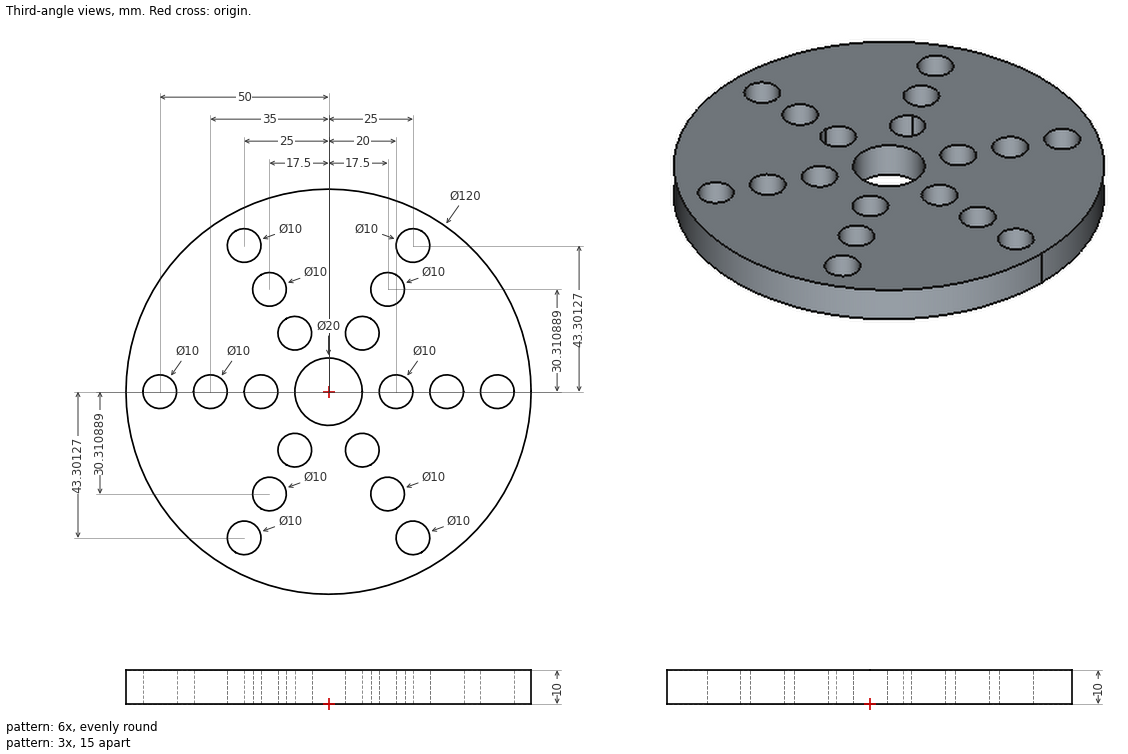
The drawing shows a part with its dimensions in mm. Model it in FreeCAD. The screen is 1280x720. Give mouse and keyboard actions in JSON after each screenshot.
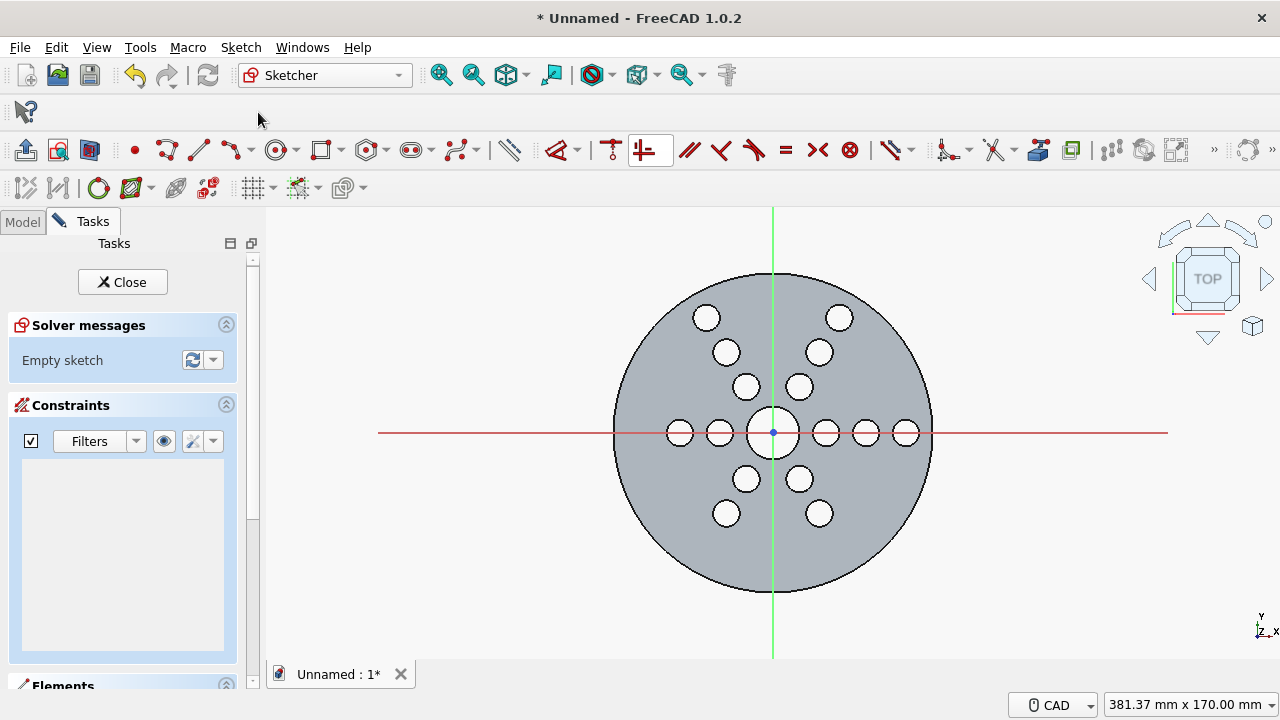
{"action": "scroll", "coordinate": [634, 433], "scroll_direction": "up", "scroll_amount": 12}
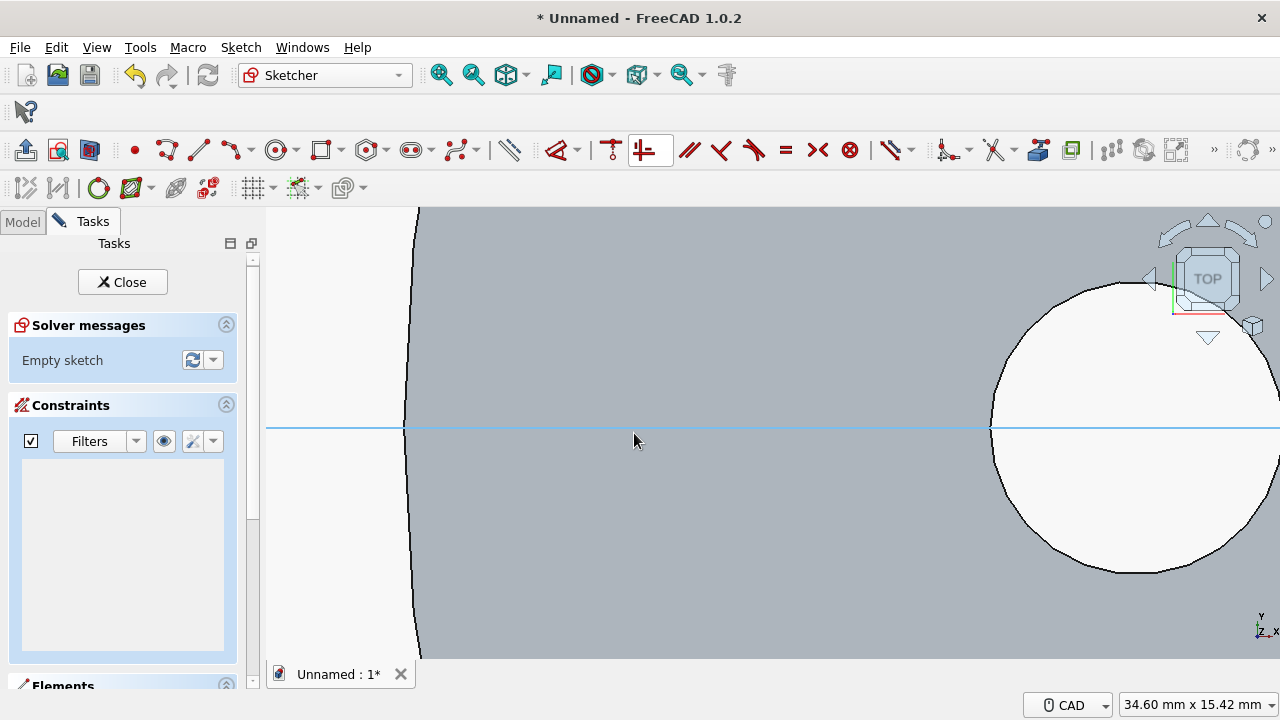
{"action": "key", "text": "g c"}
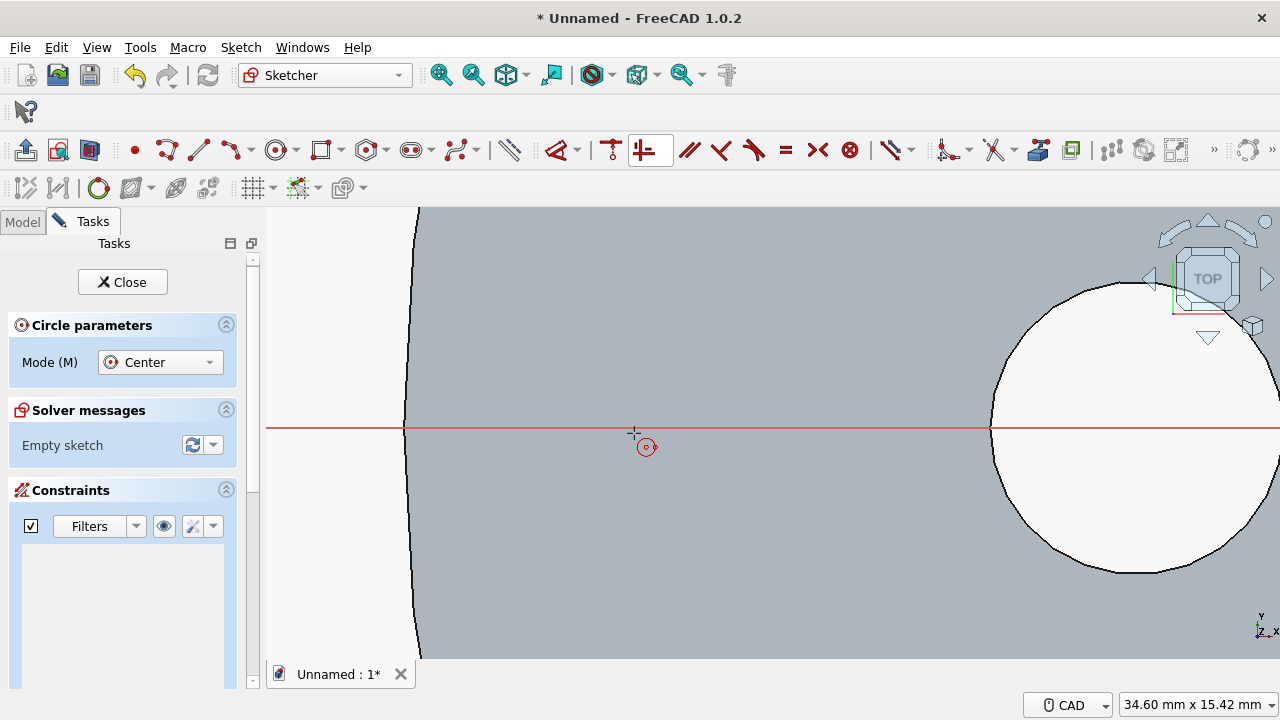
{"action": "left_click", "coordinate": [697, 428]}
{"action": "left_click", "coordinate": [801, 324]}
{"action": "key", "text": "Escape"}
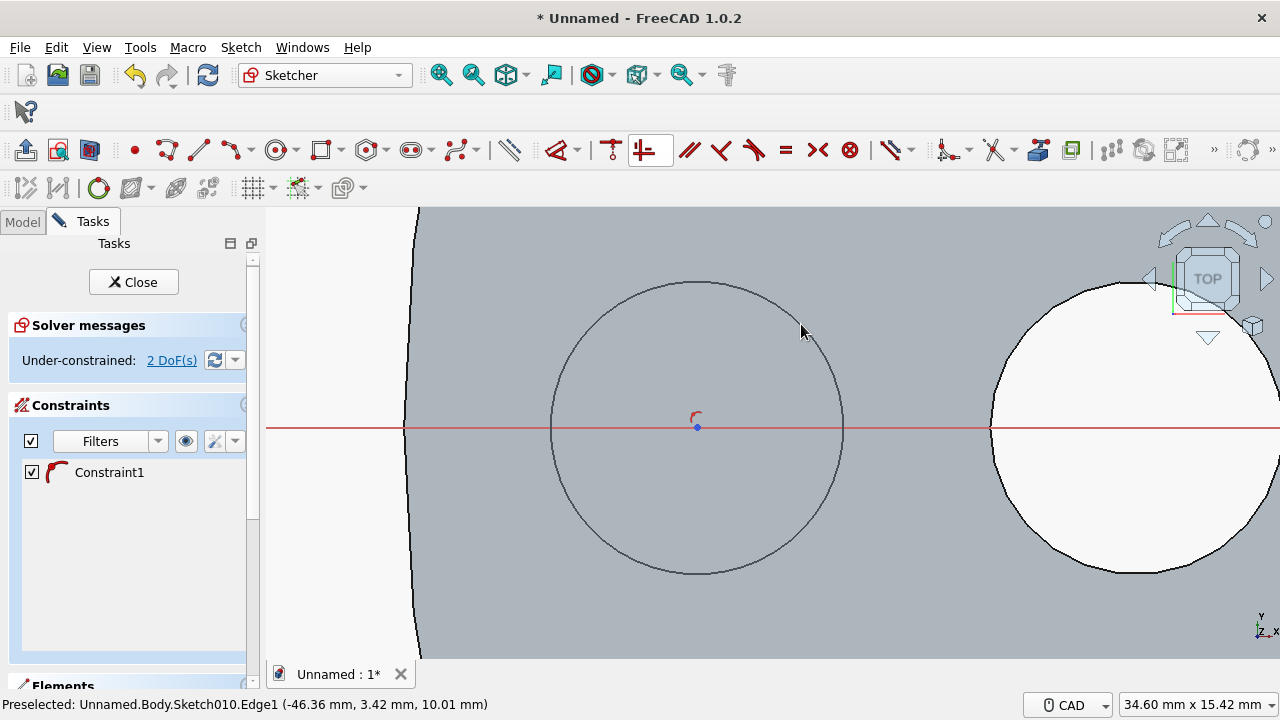
{"action": "left_click", "coordinate": [556, 150]}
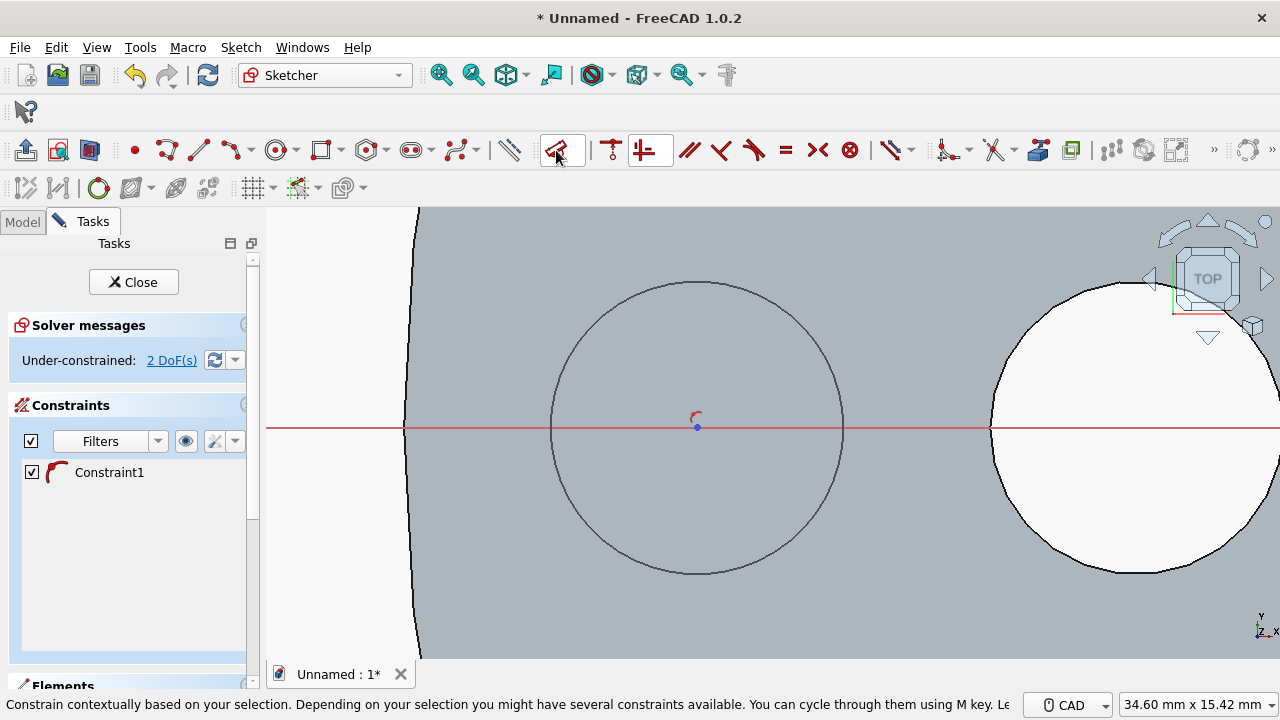
{"action": "left_click", "coordinate": [800, 324]}
{"action": "left_click", "coordinate": [823, 301]}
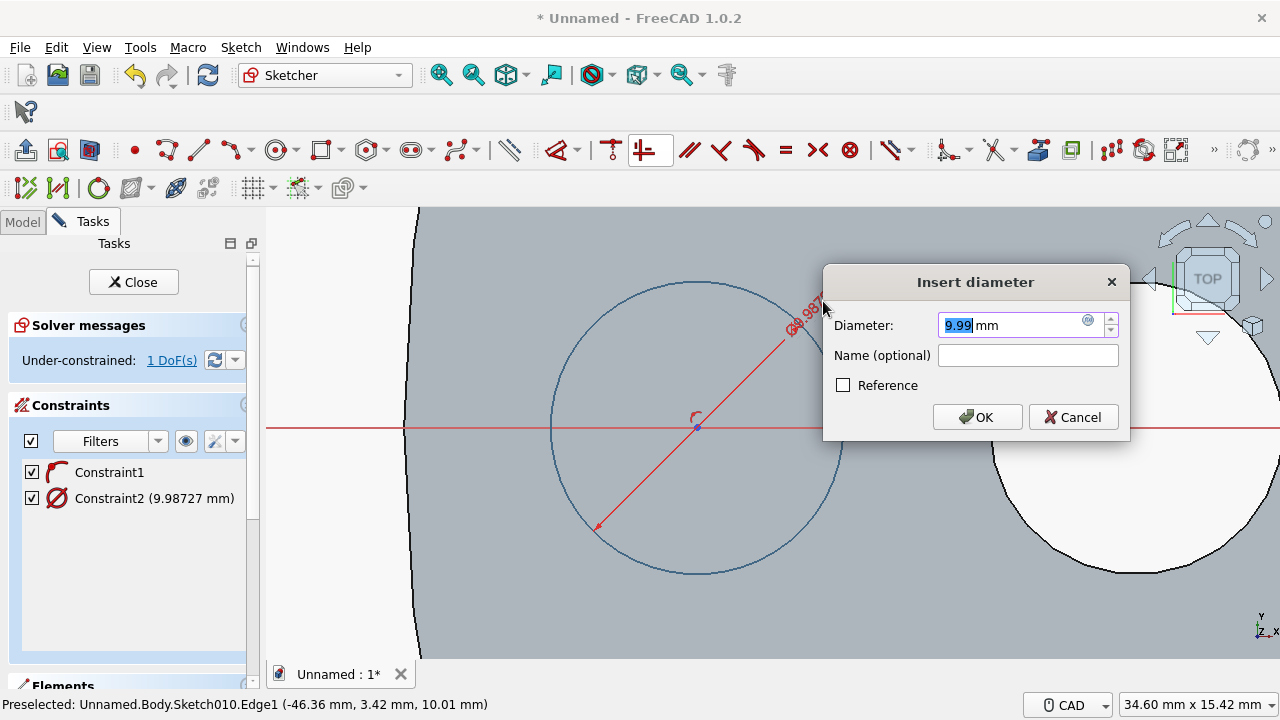
{"action": "type", "text": "10"}
{"action": "key", "text": "Return"}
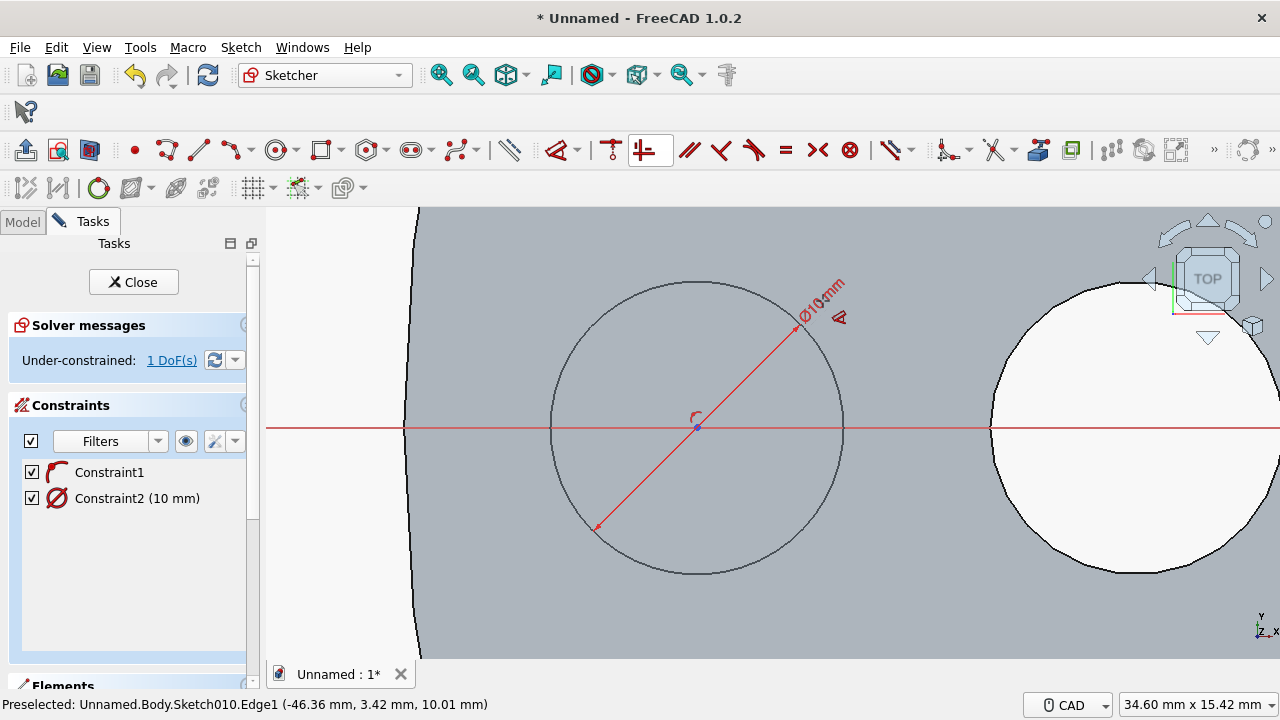
{"action": "left_click", "coordinate": [697, 428]}
{"action": "left_click", "coordinate": [906, 462]}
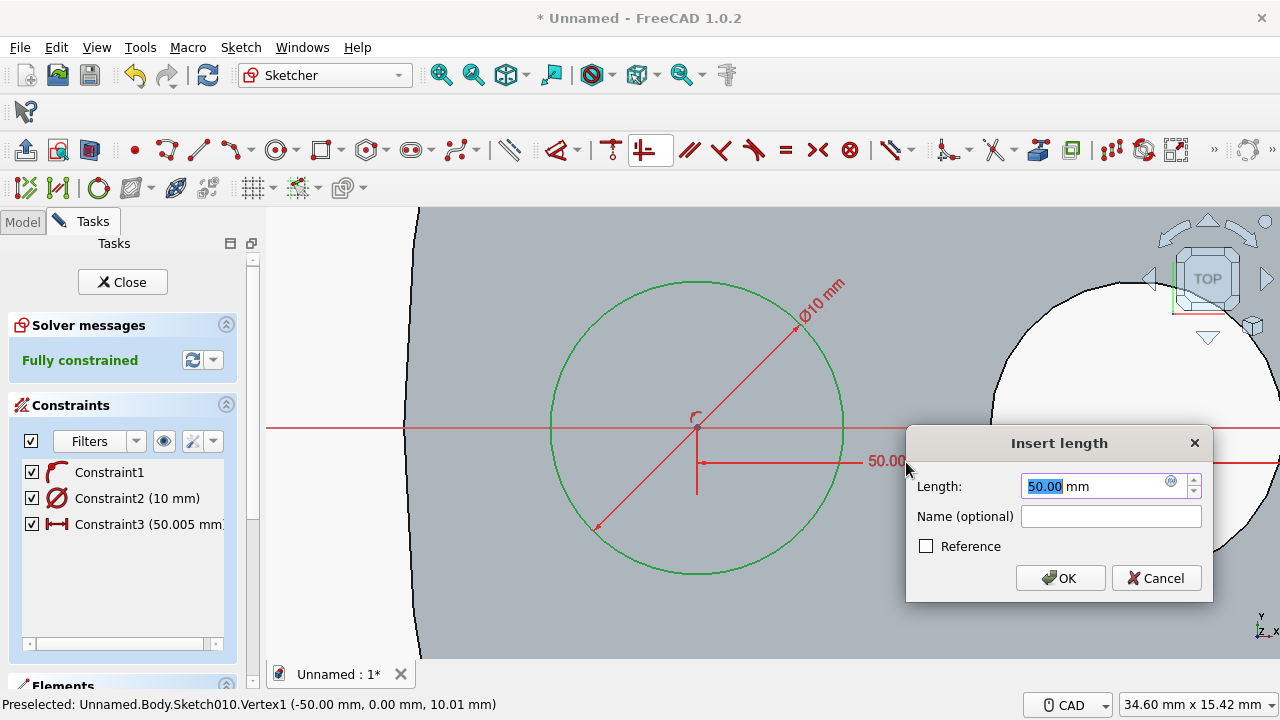
{"action": "type", "text": "50"}
{"action": "key", "text": "Return"}
{"action": "key", "text": "Escape"}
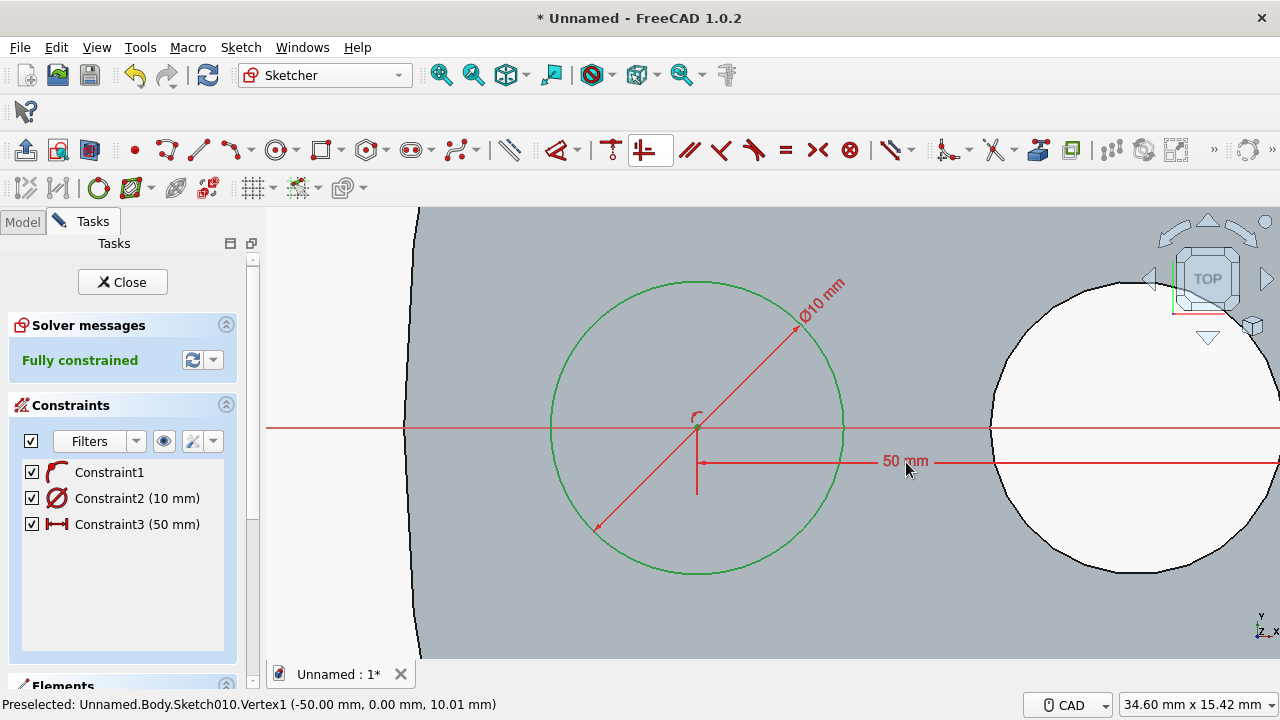
{"action": "left_click", "coordinate": [123, 282]}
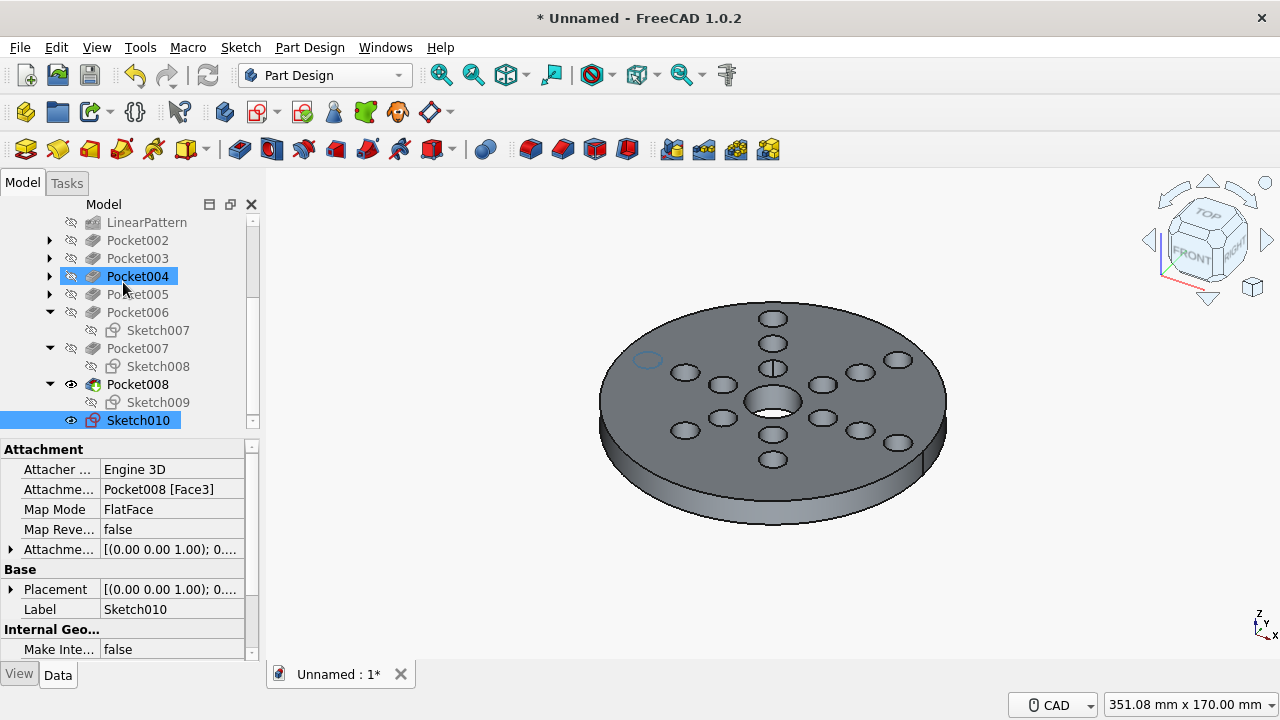
{"action": "left_click", "coordinate": [240, 150]}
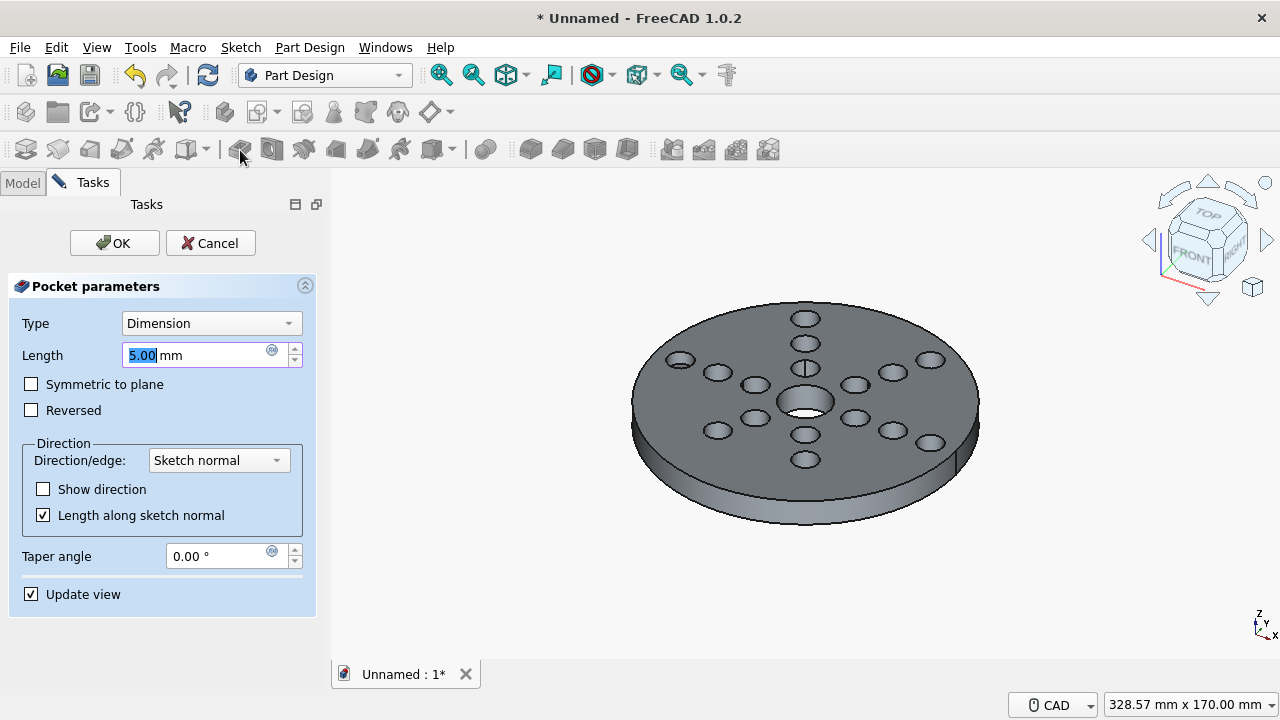
{"action": "type", "text": "10"}
{"action": "key", "text": "Tab"}